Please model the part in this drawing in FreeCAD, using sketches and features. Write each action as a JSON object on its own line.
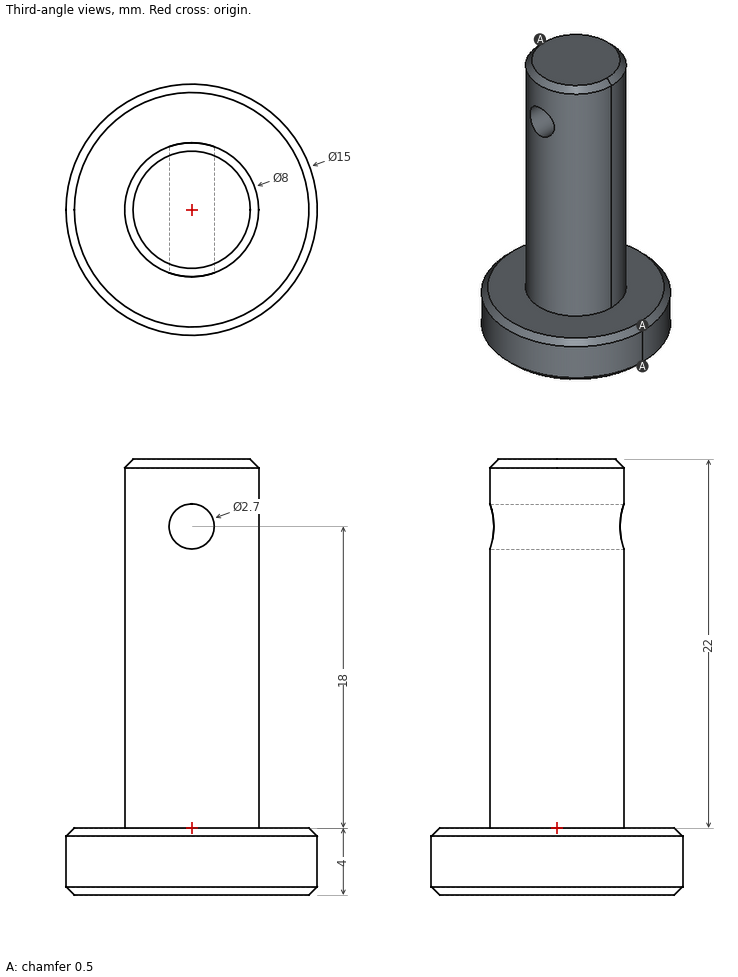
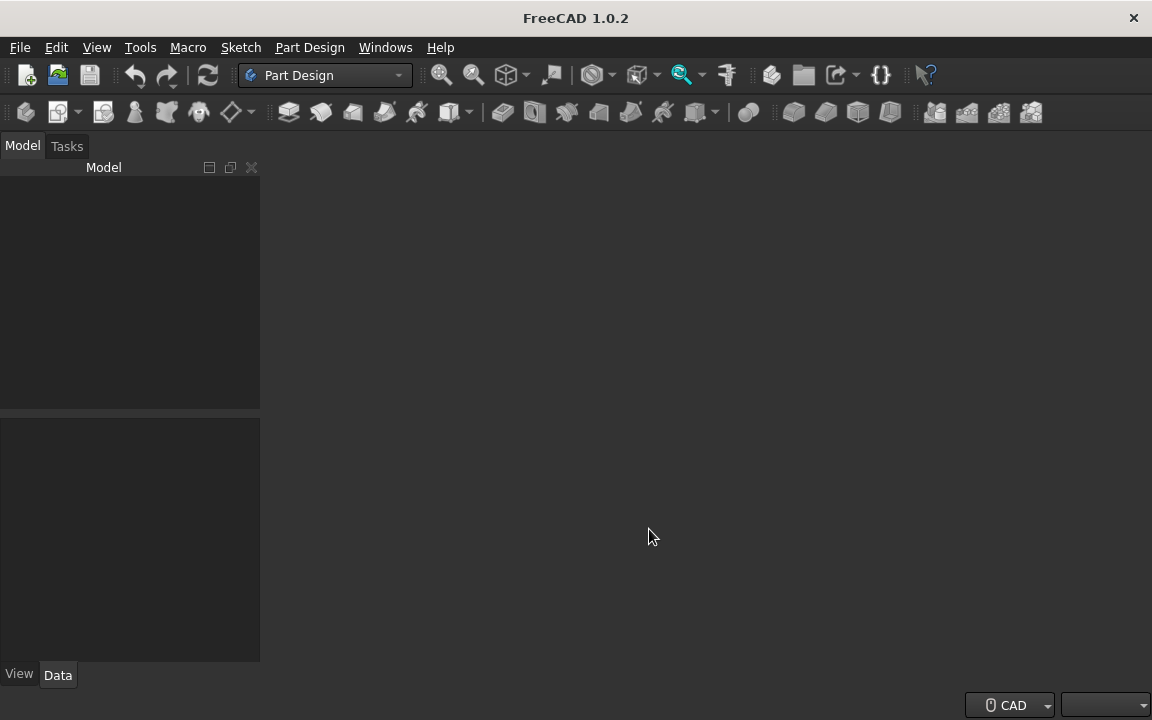
{"action": "left_click", "coordinate": [26, 76]}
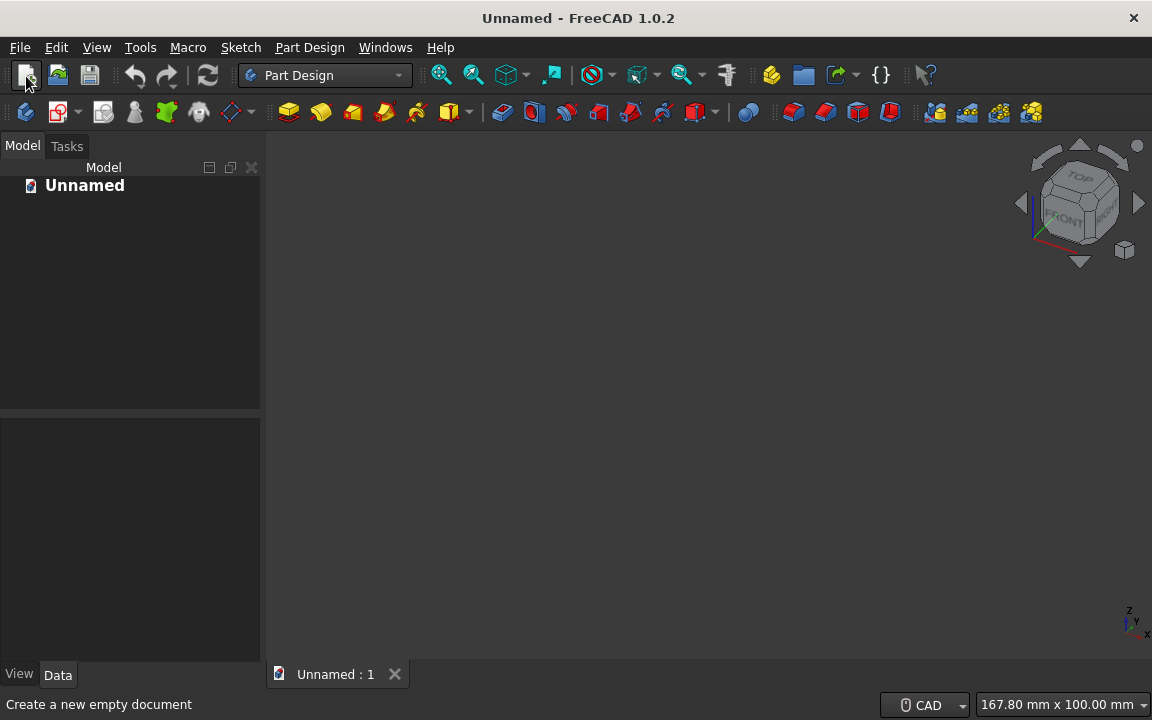
{"action": "left_click", "coordinate": [58, 112]}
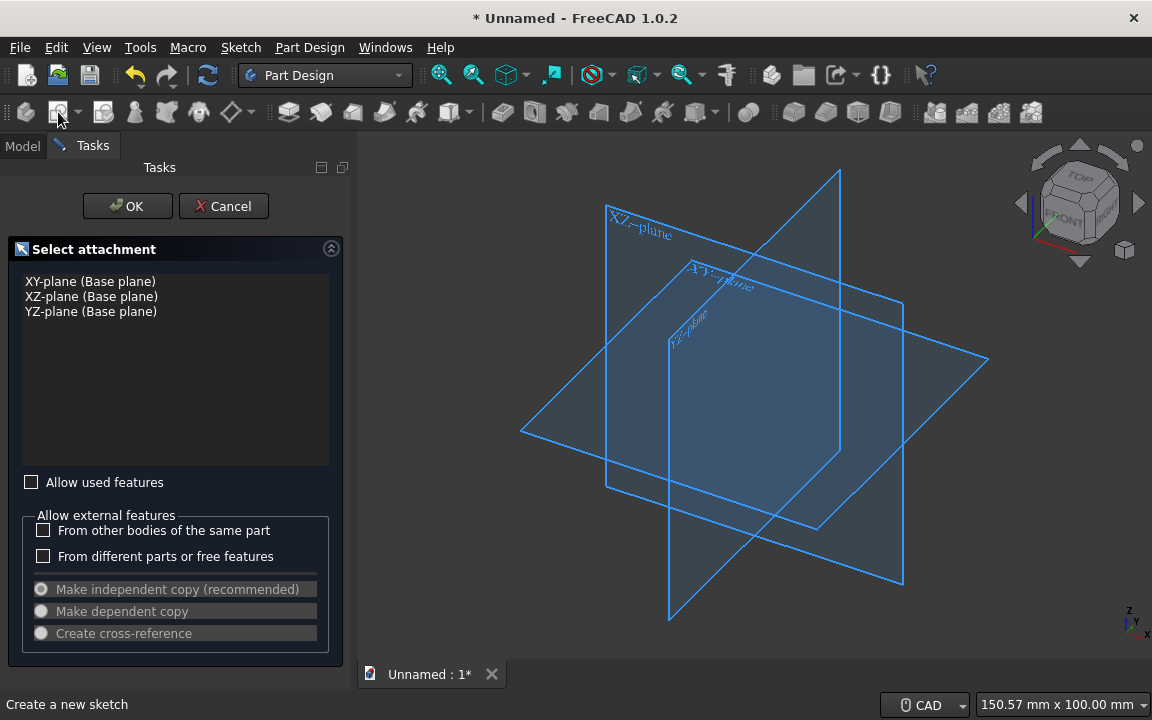
{"action": "left_click", "coordinate": [82, 282]}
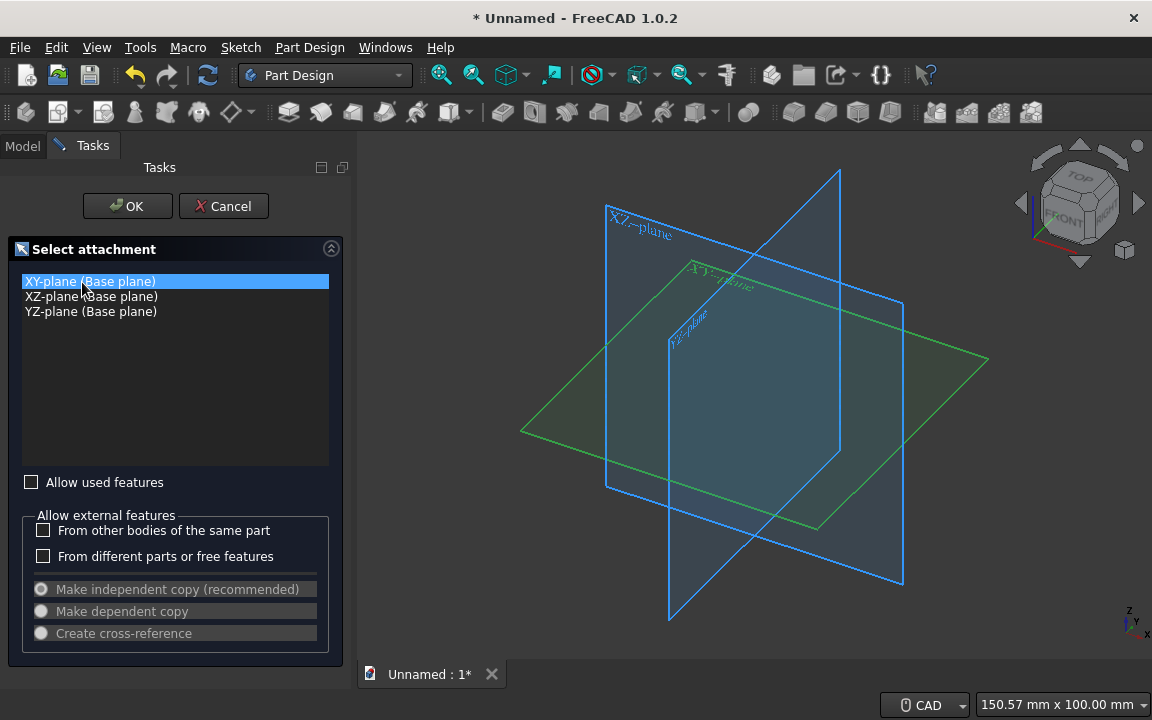
{"action": "left_click", "coordinate": [128, 206]}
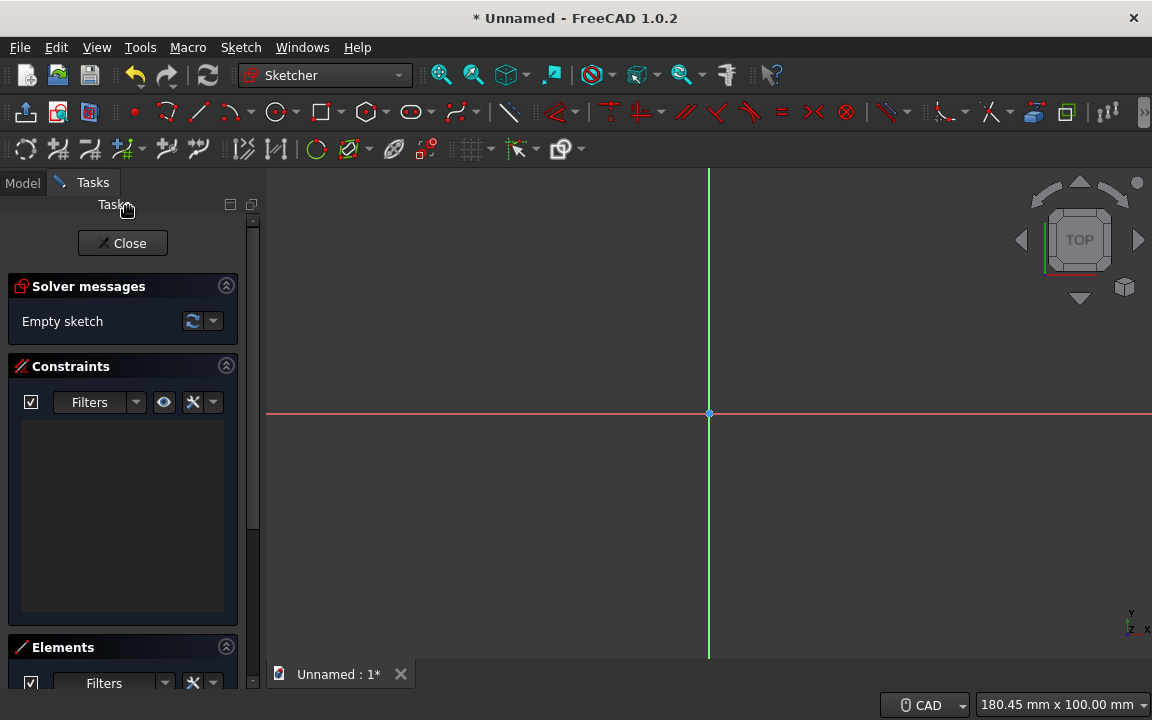
{"action": "scroll", "coordinate": [720, 414], "scroll_direction": "up", "scroll_amount": 10}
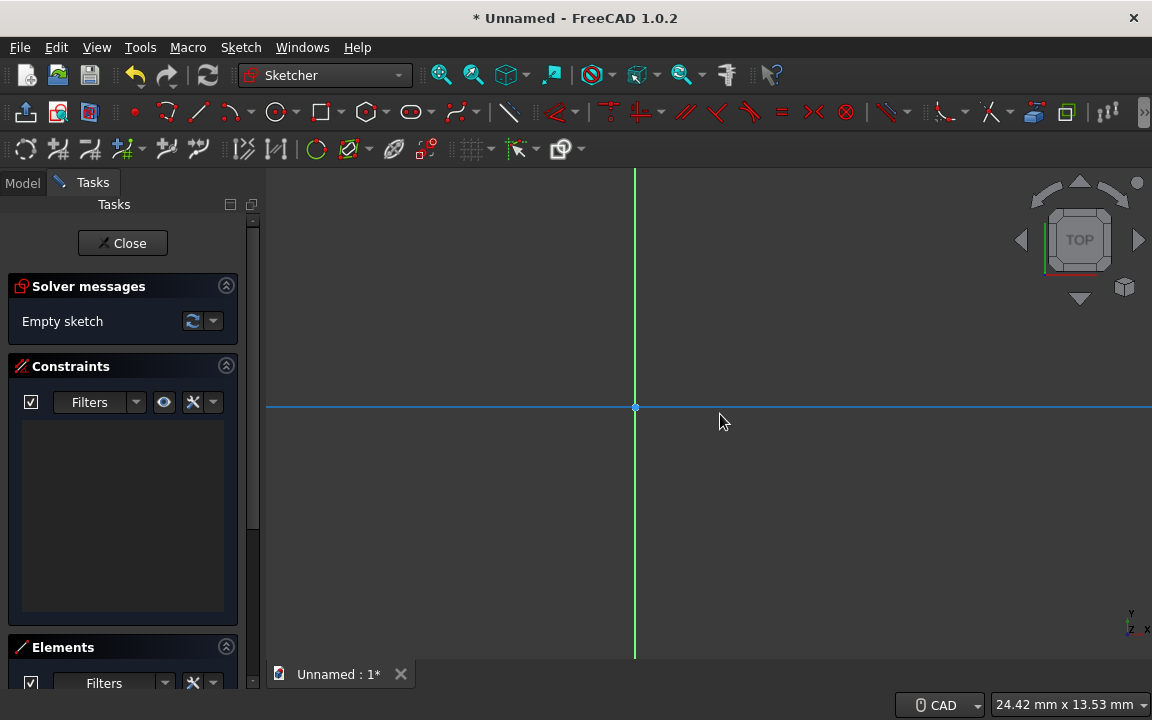
{"action": "left_click", "coordinate": [276, 112]}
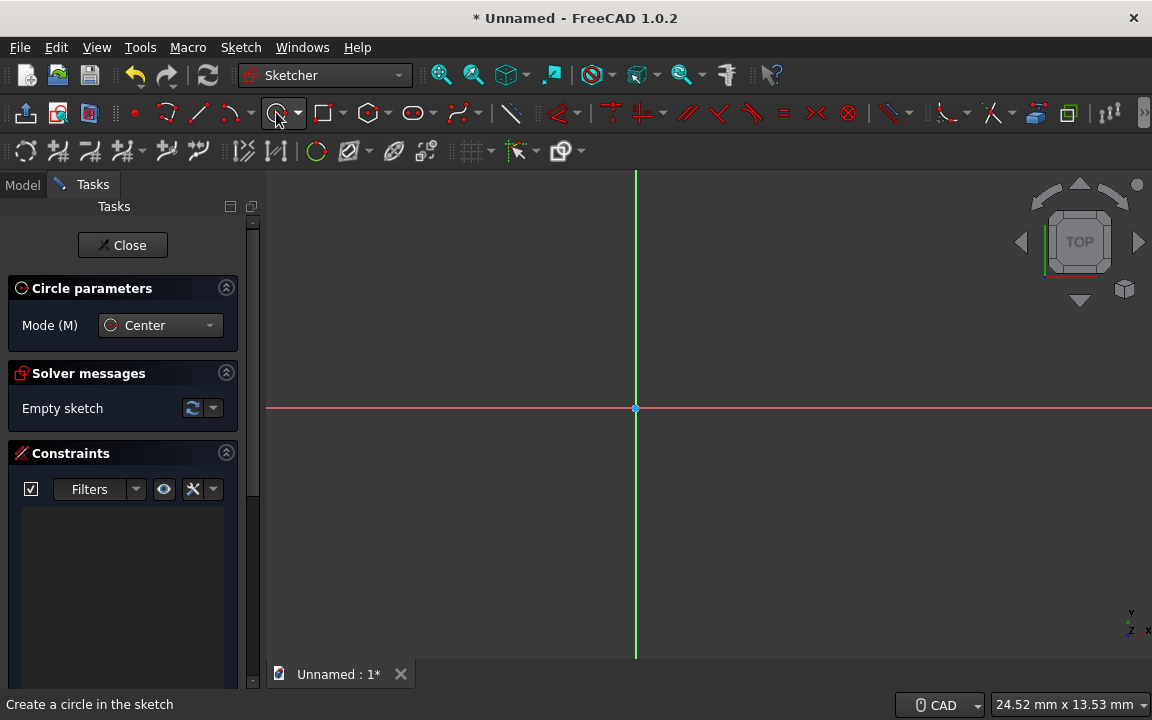
{"action": "left_click", "coordinate": [636, 408]}
{"action": "left_click", "coordinate": [738, 306]}
{"action": "key", "text": "Escape"}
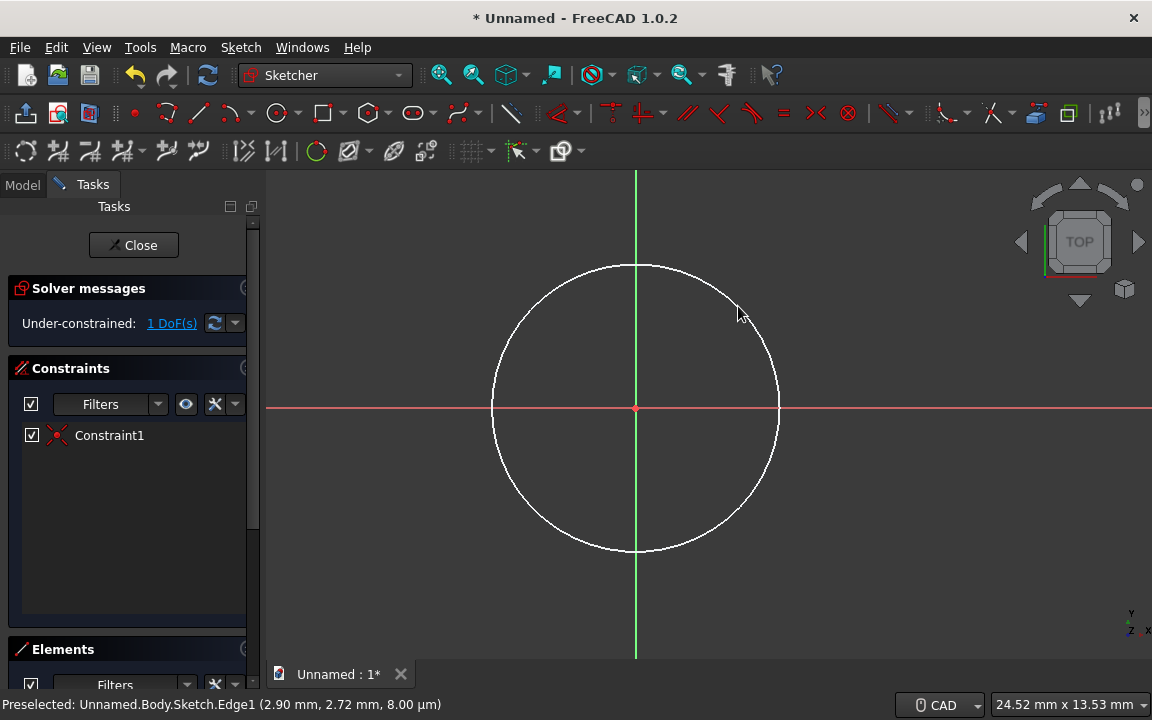
{"action": "left_click", "coordinate": [737, 306]}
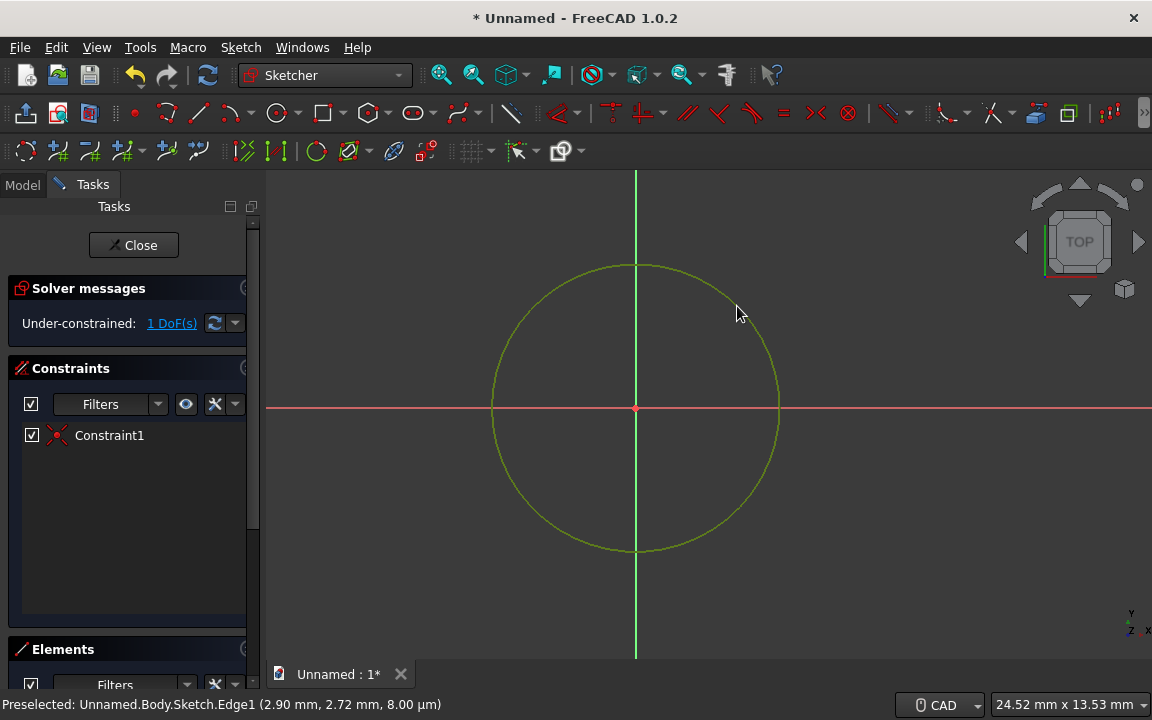
{"action": "left_click", "coordinate": [580, 114]}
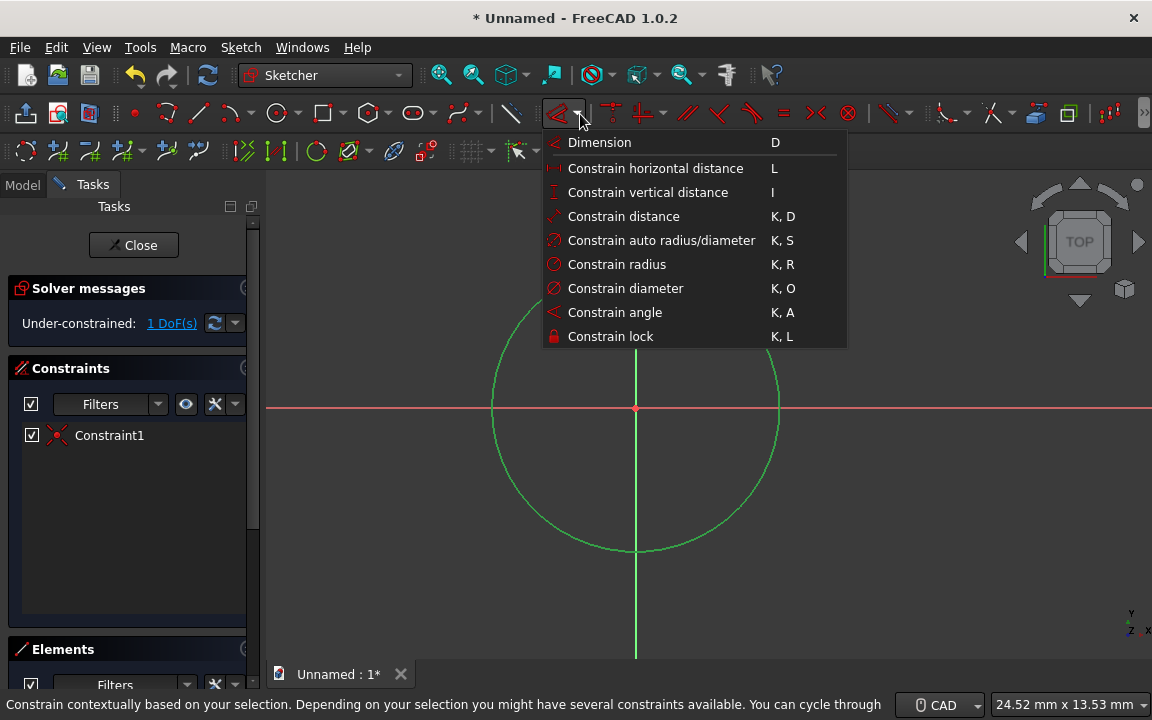
{"action": "left_click", "coordinate": [695, 288]}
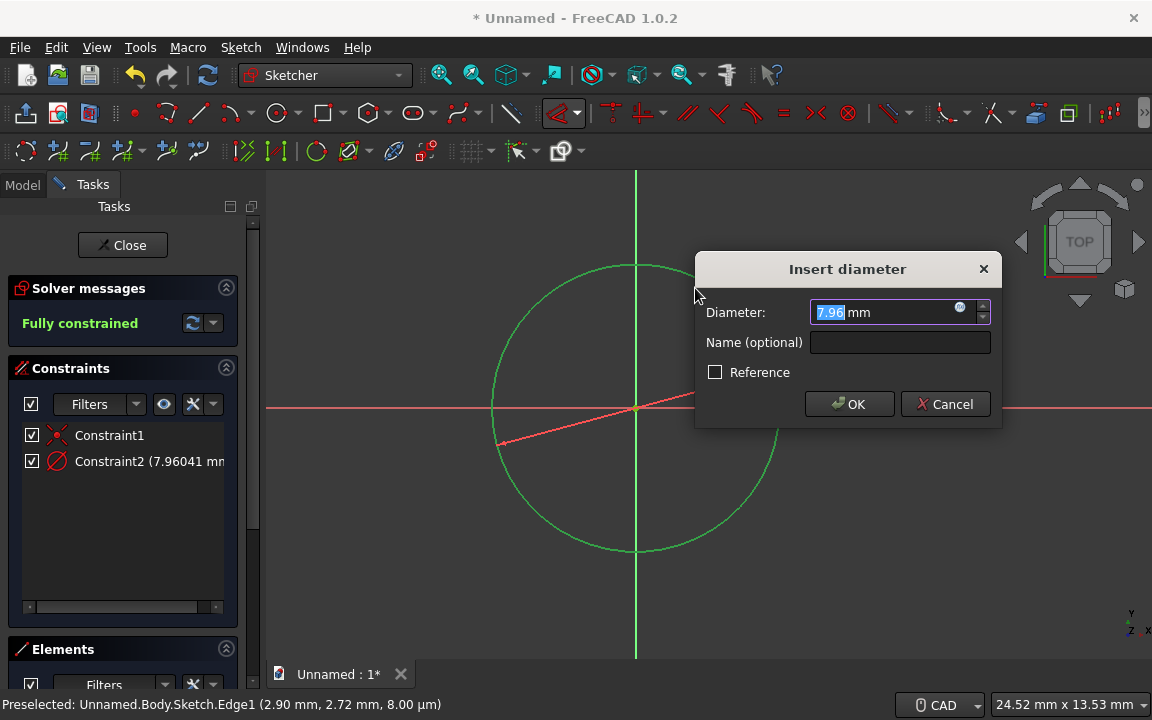
{"action": "type", "text": "8"}
{"action": "key", "text": "Return"}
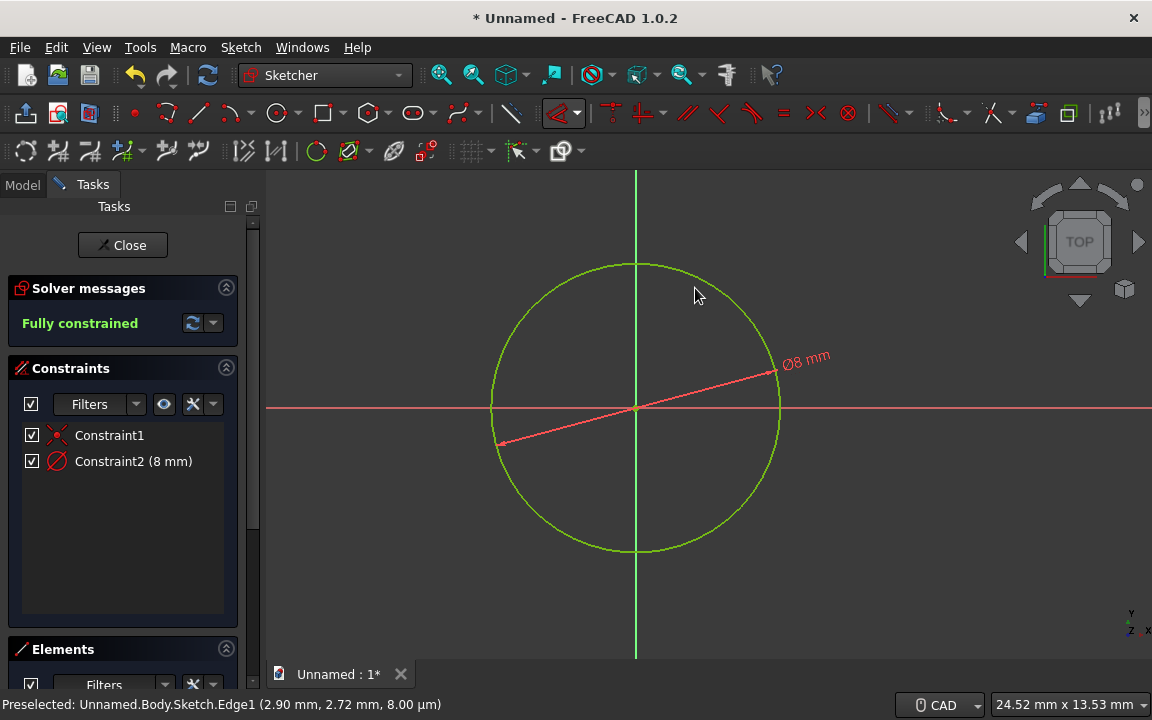
{"action": "left_click", "coordinate": [123, 245]}